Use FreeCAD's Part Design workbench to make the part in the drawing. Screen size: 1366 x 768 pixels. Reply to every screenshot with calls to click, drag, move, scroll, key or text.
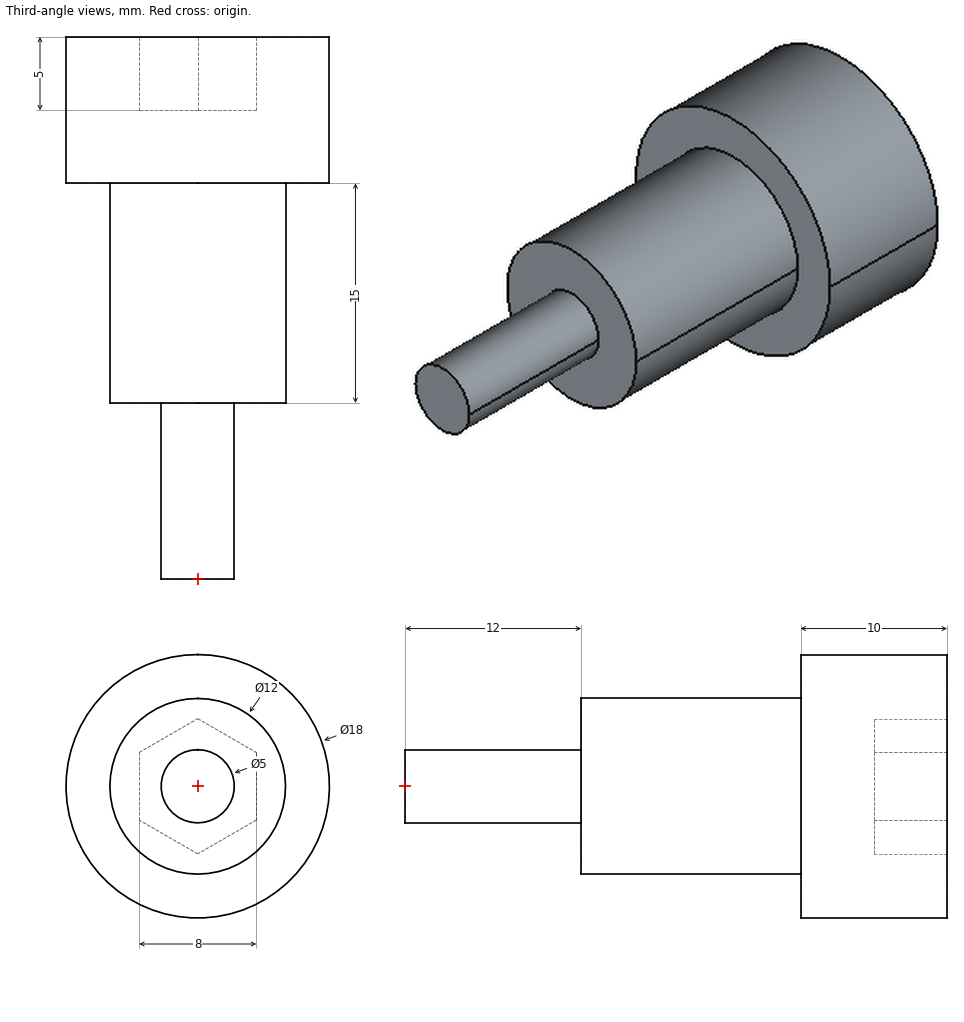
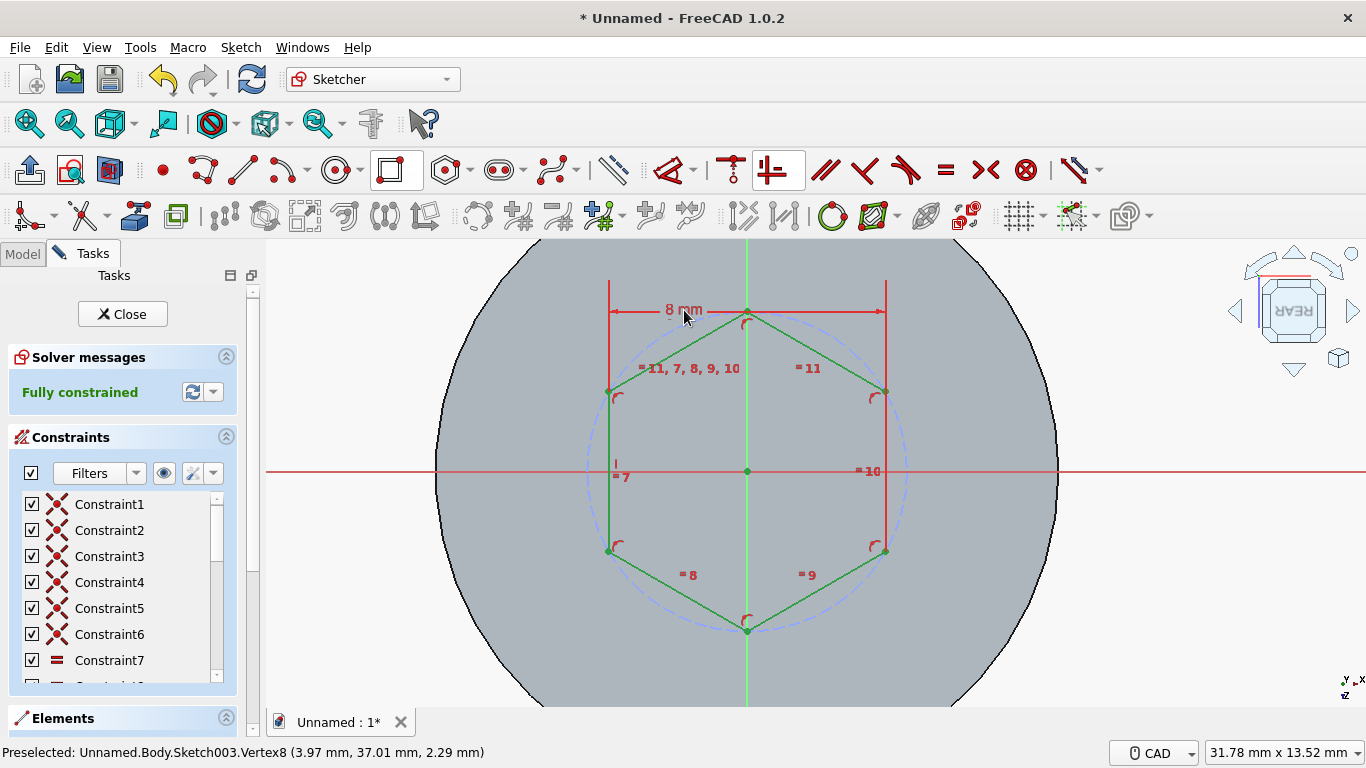
click(123, 314)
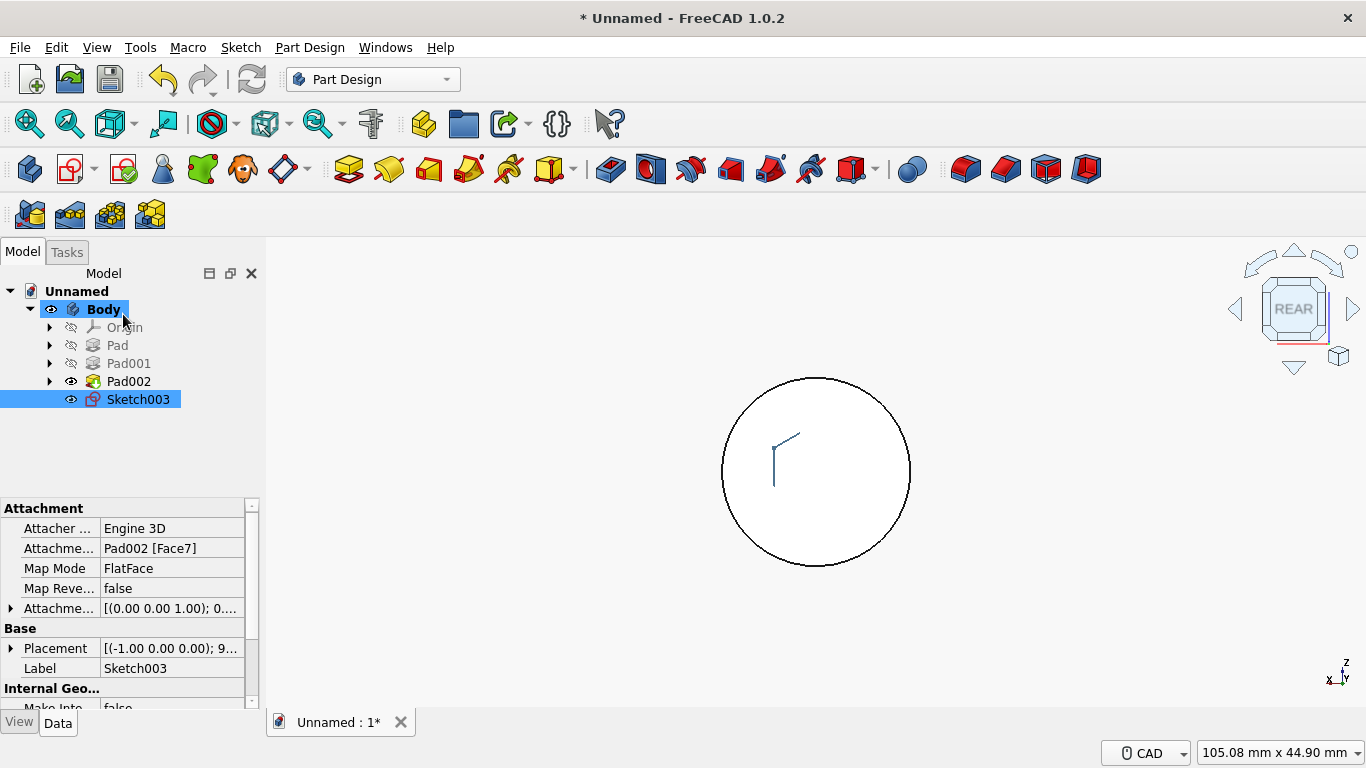
click(612, 170)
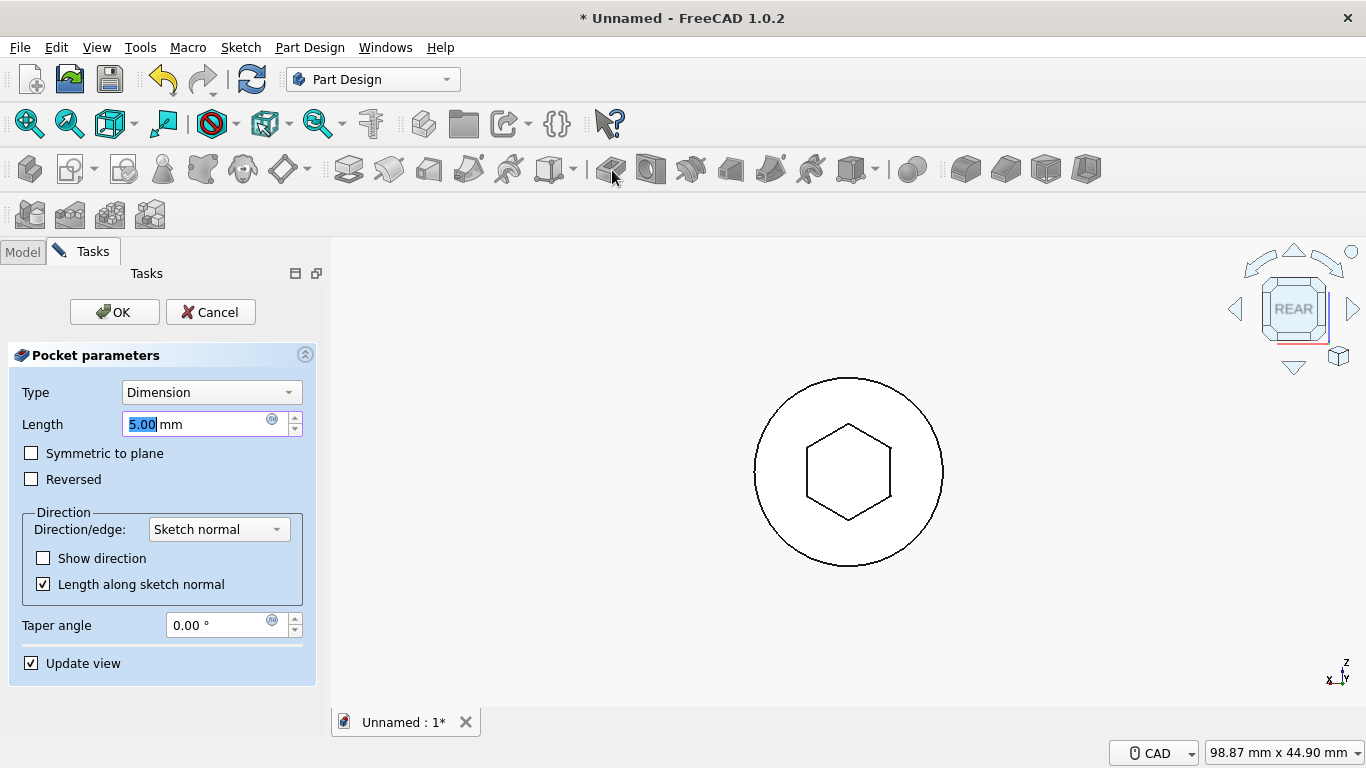
text(5)
key(Tab)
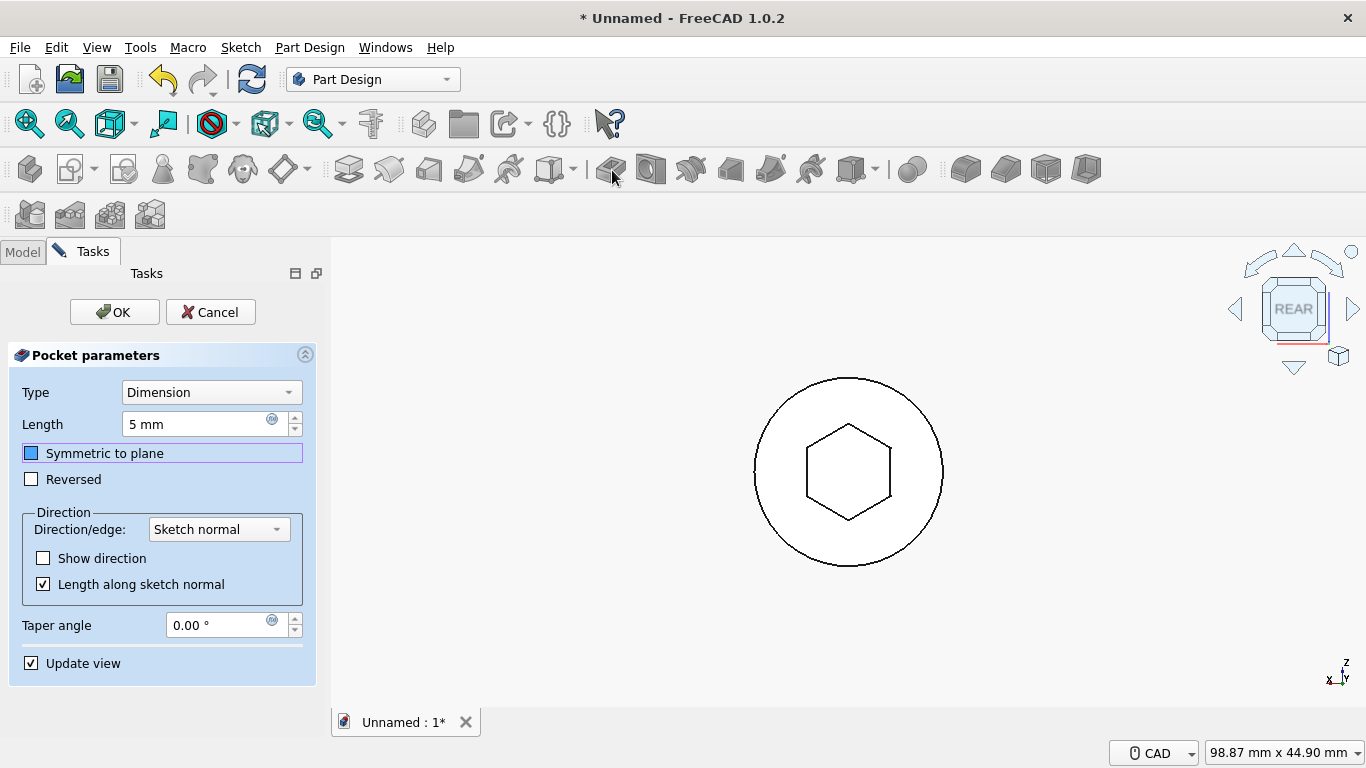
click(115, 312)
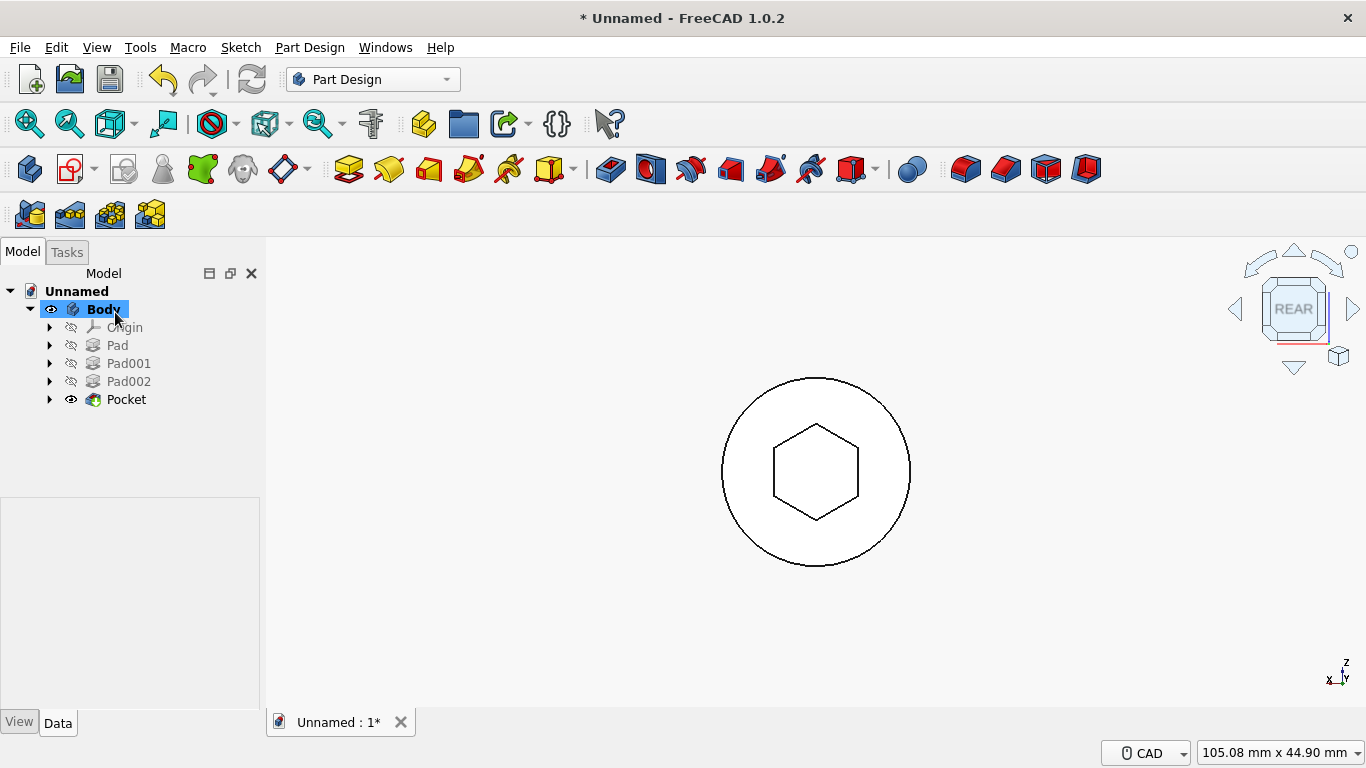
key(0)